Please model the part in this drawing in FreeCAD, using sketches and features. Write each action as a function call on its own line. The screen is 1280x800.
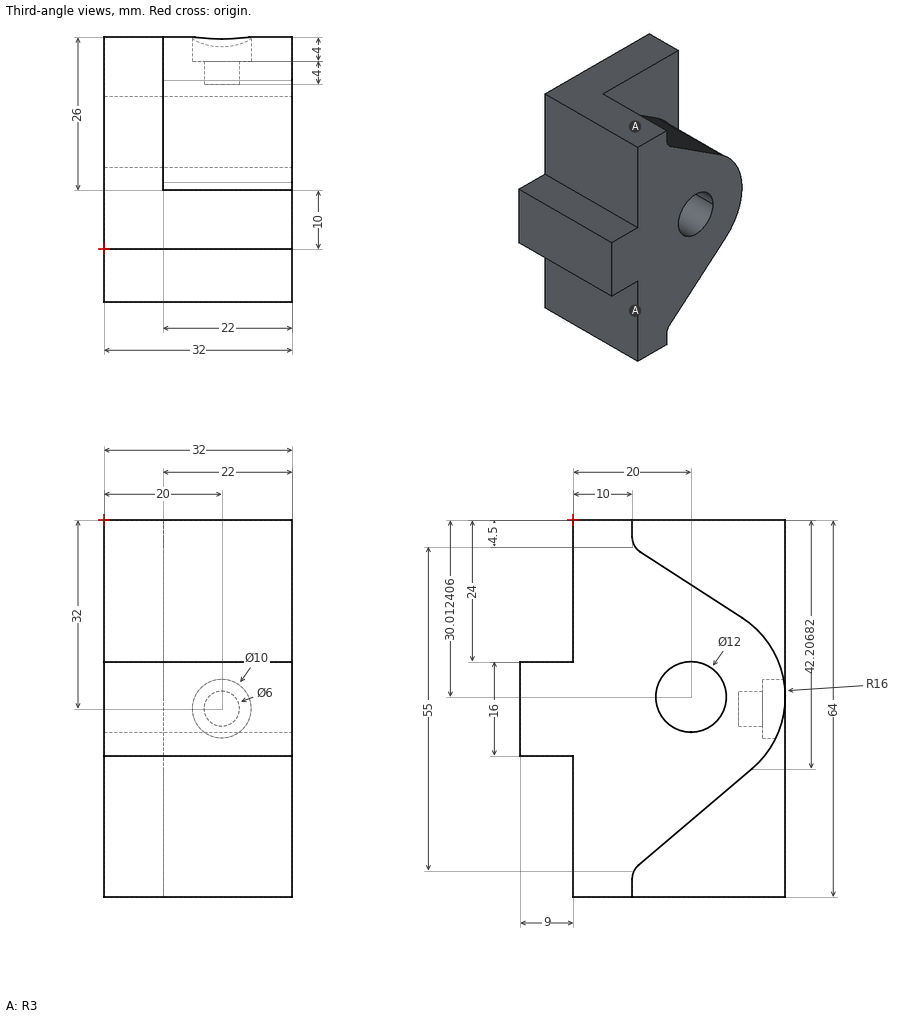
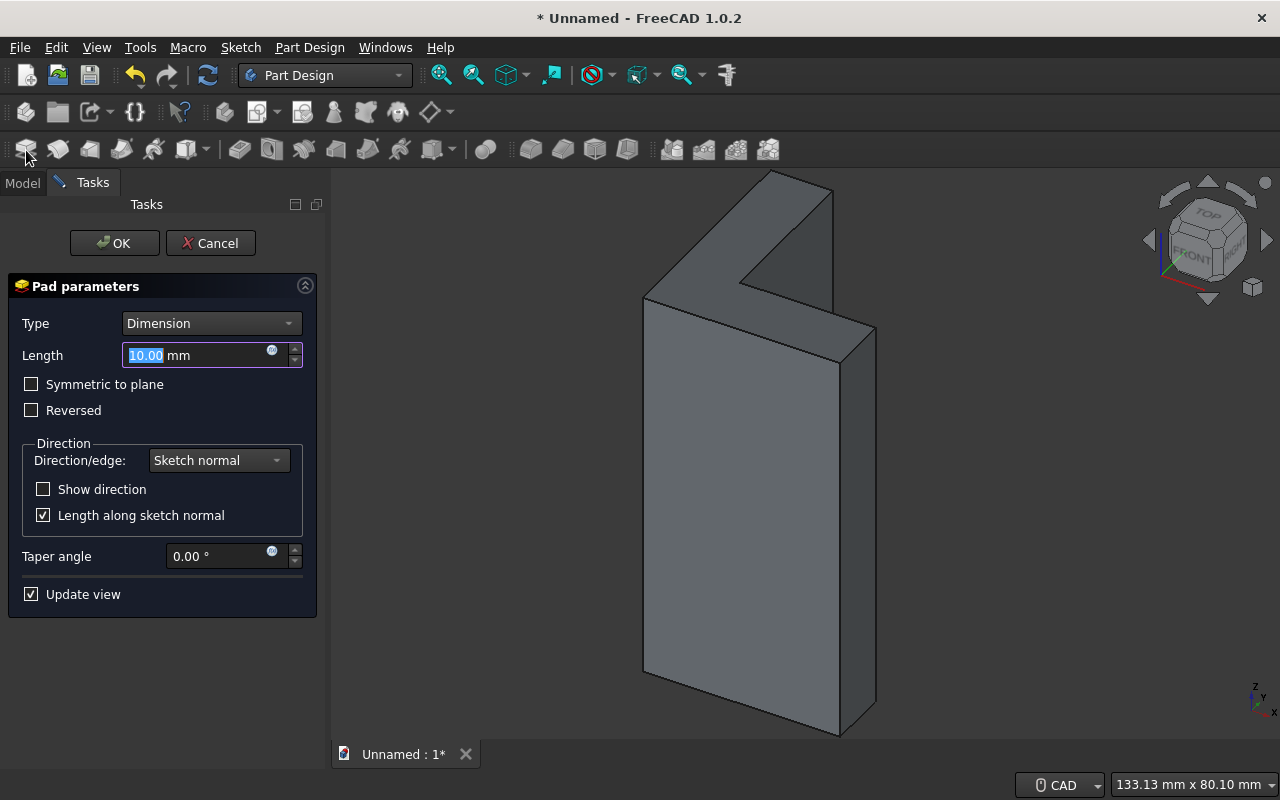
text(22)
key(Tab)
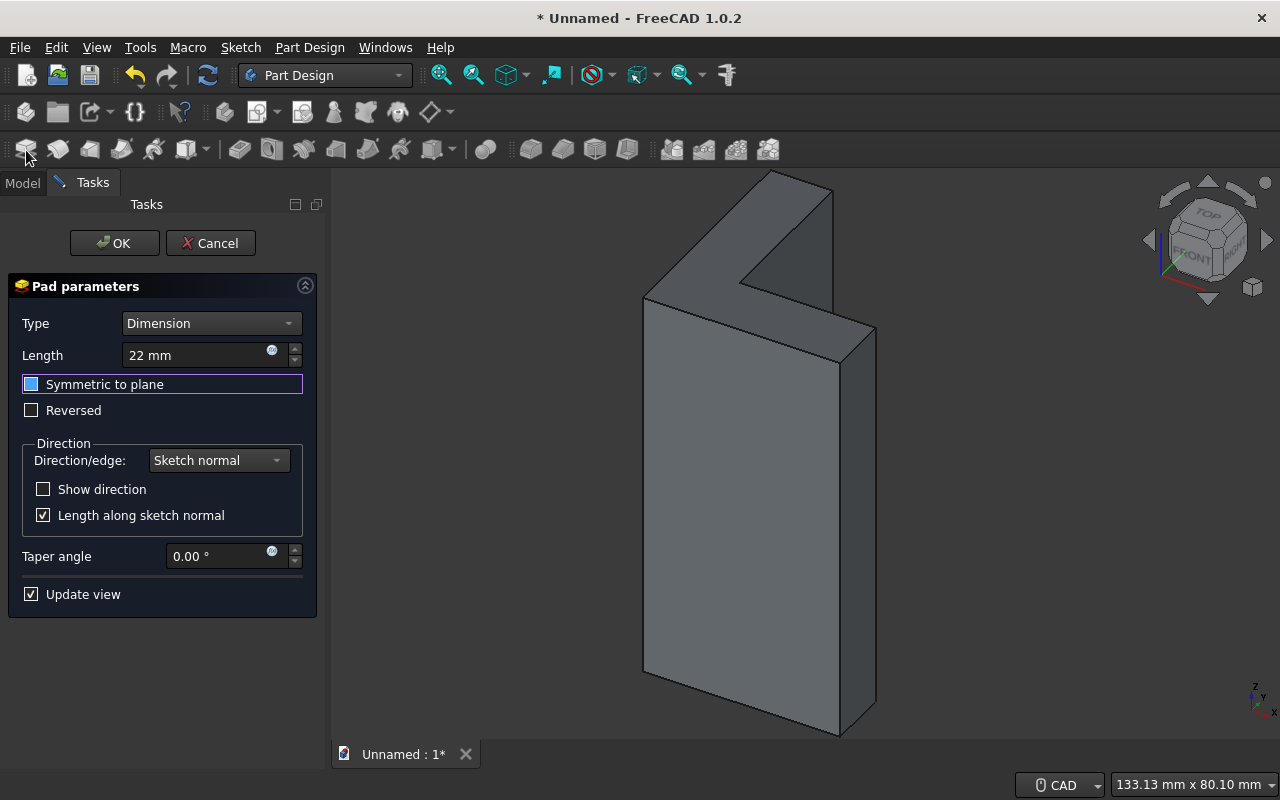
click(30, 410)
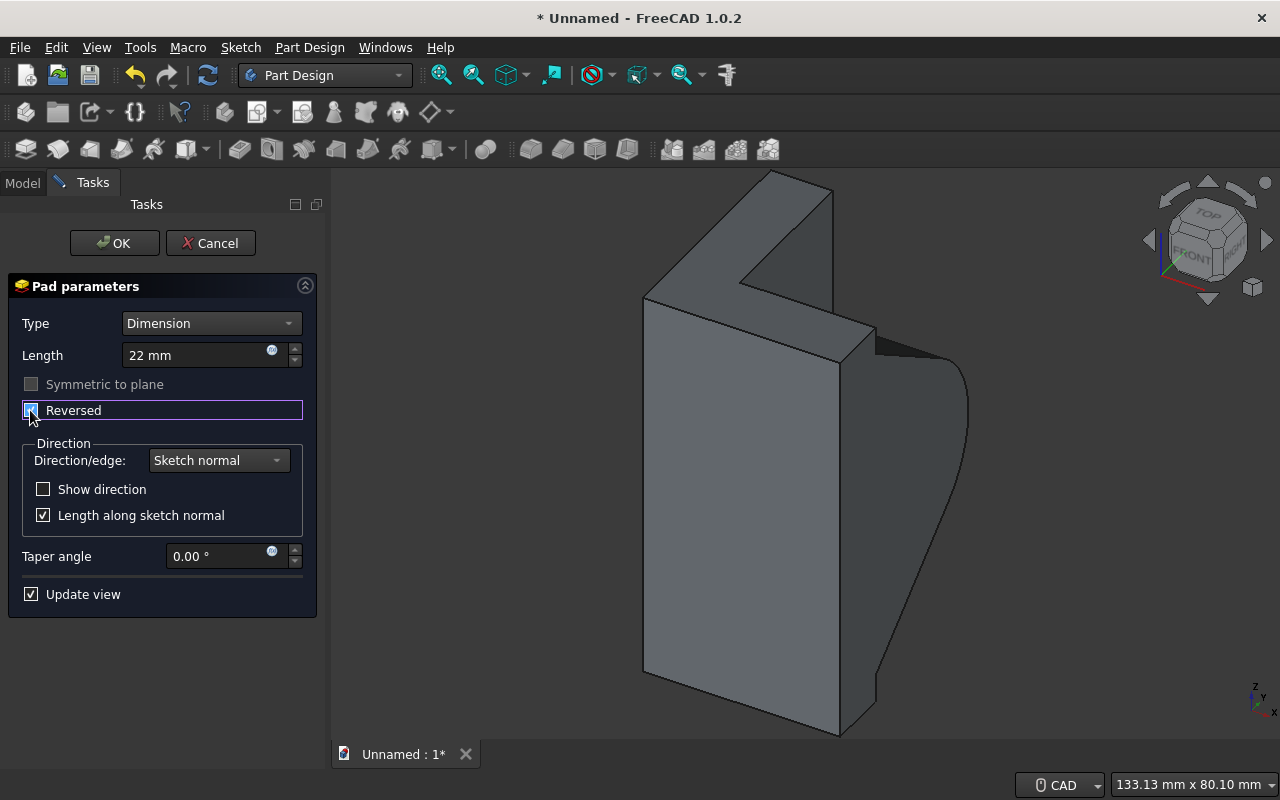
click(115, 243)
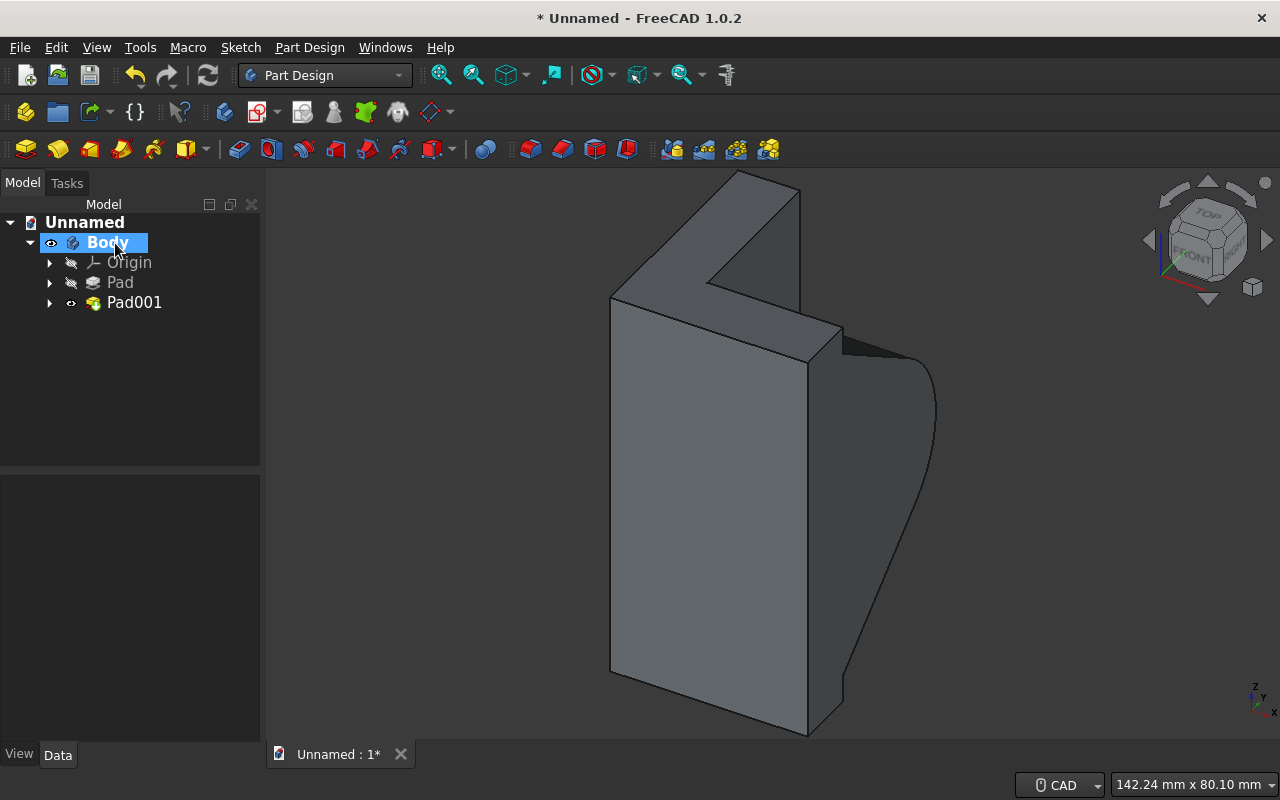
click(872, 485)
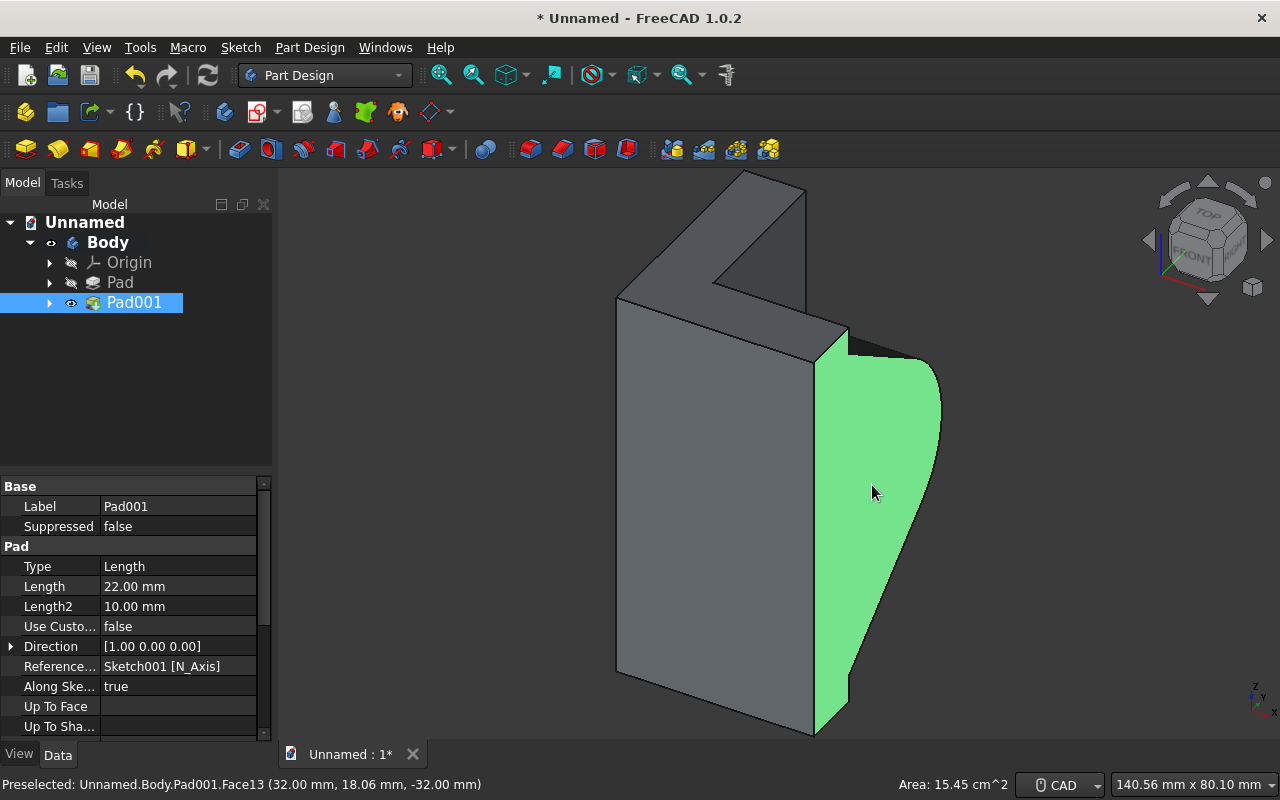
click(258, 112)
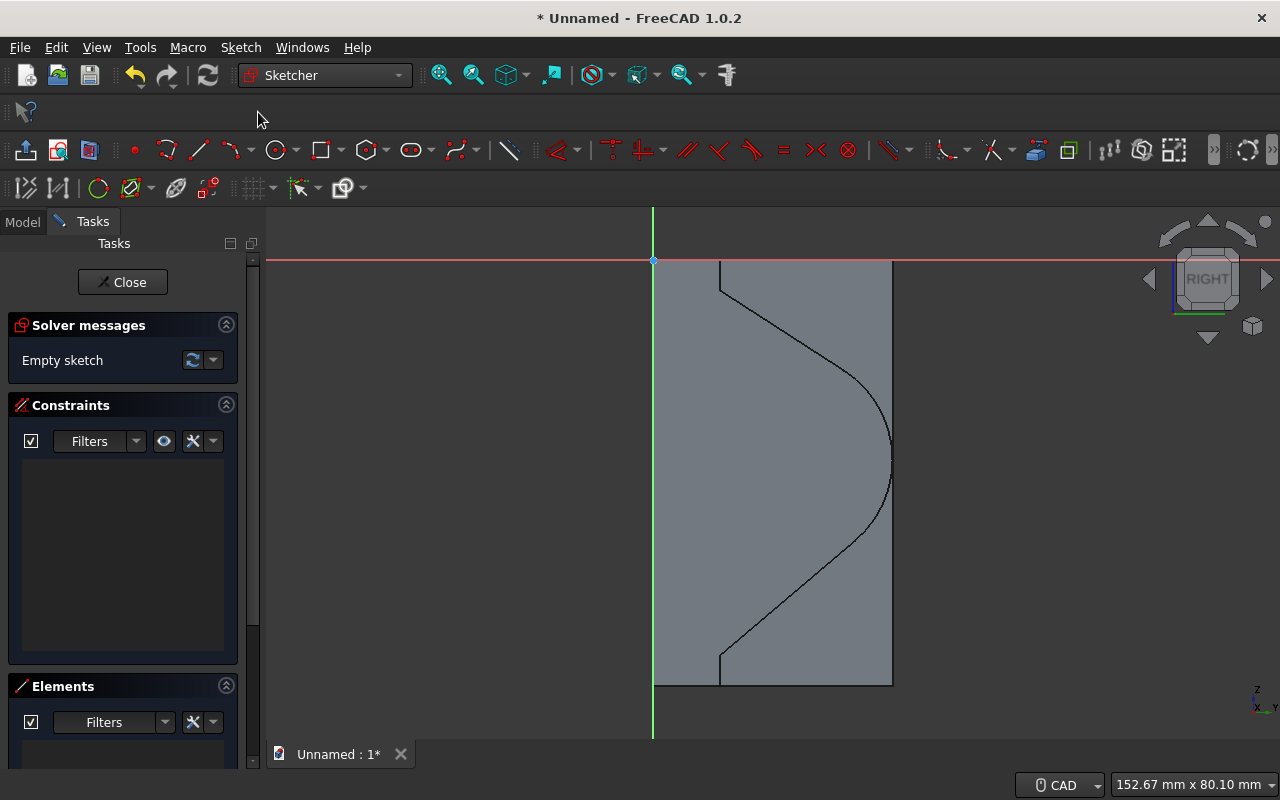
scroll(813, 455, up, 7)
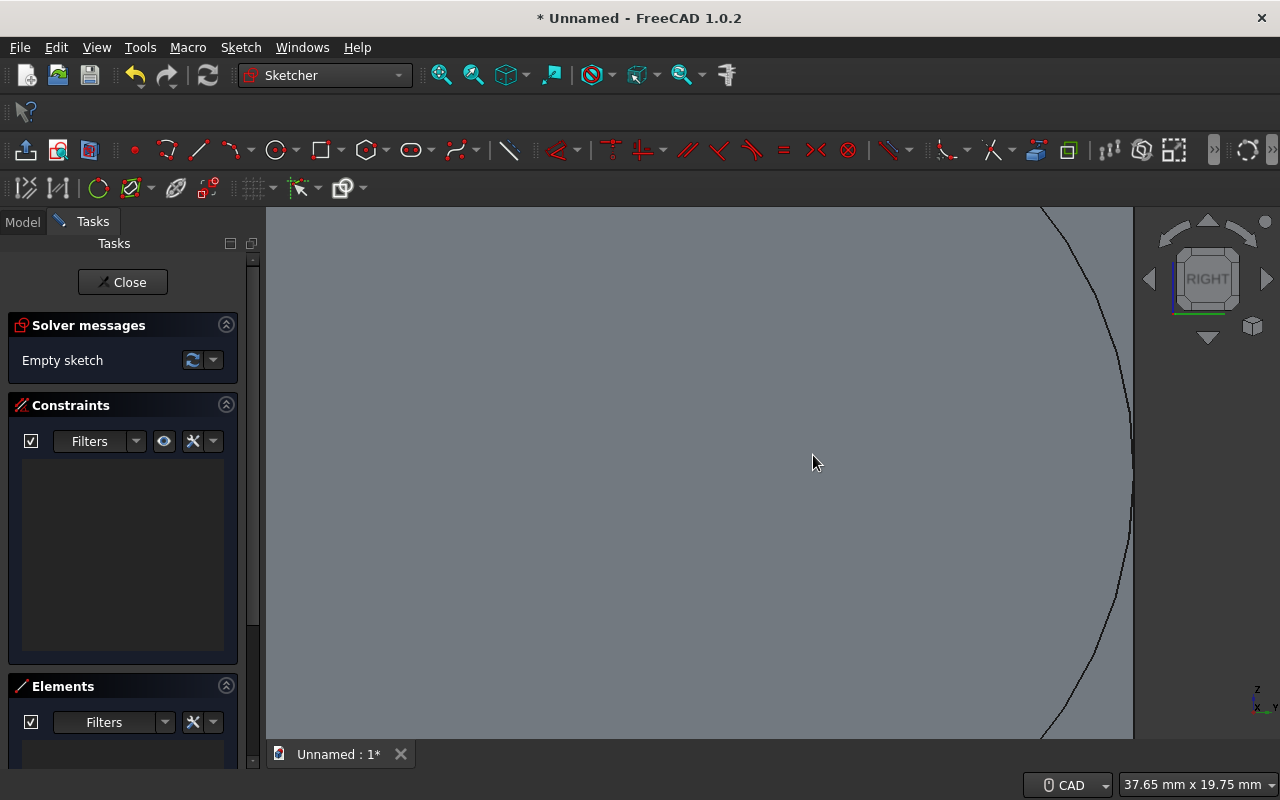
key(g)
key(c)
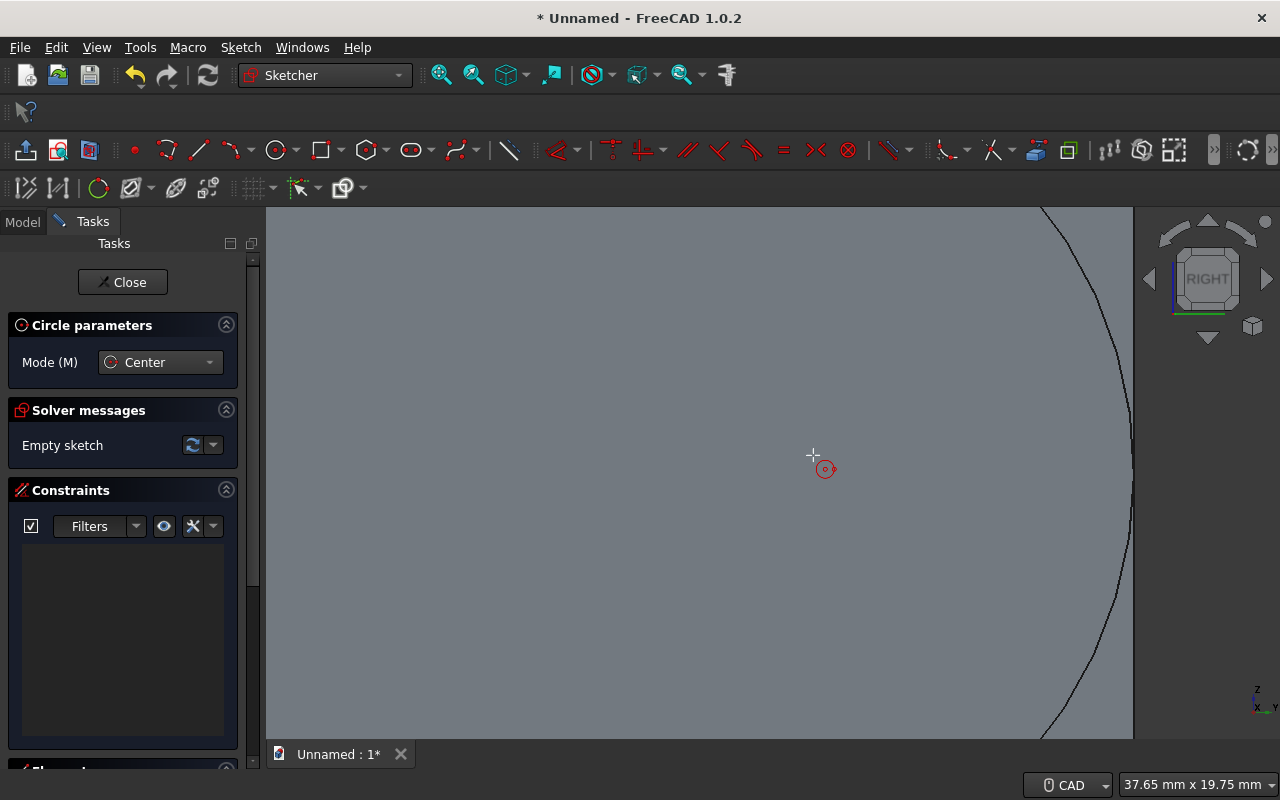
click(703, 473)
move(817, 359)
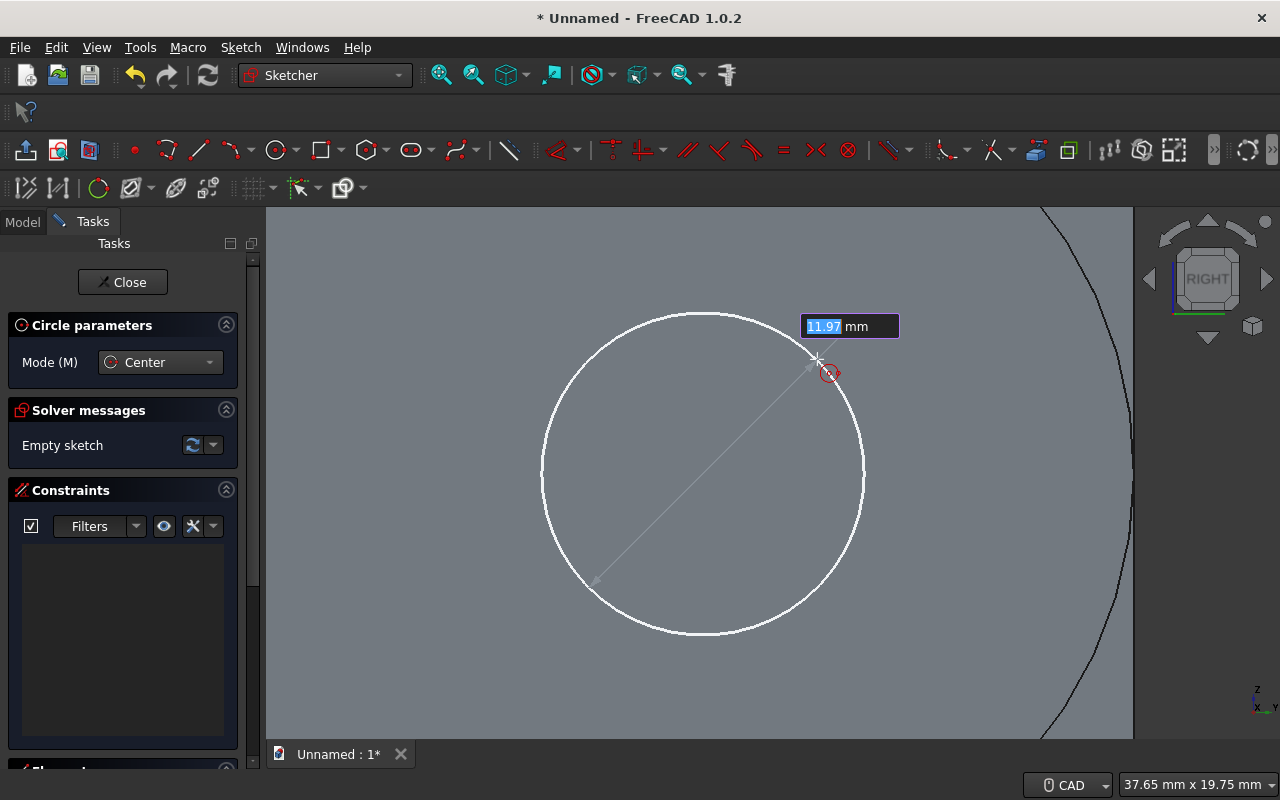
text(12)
key(Return)
key(Escape)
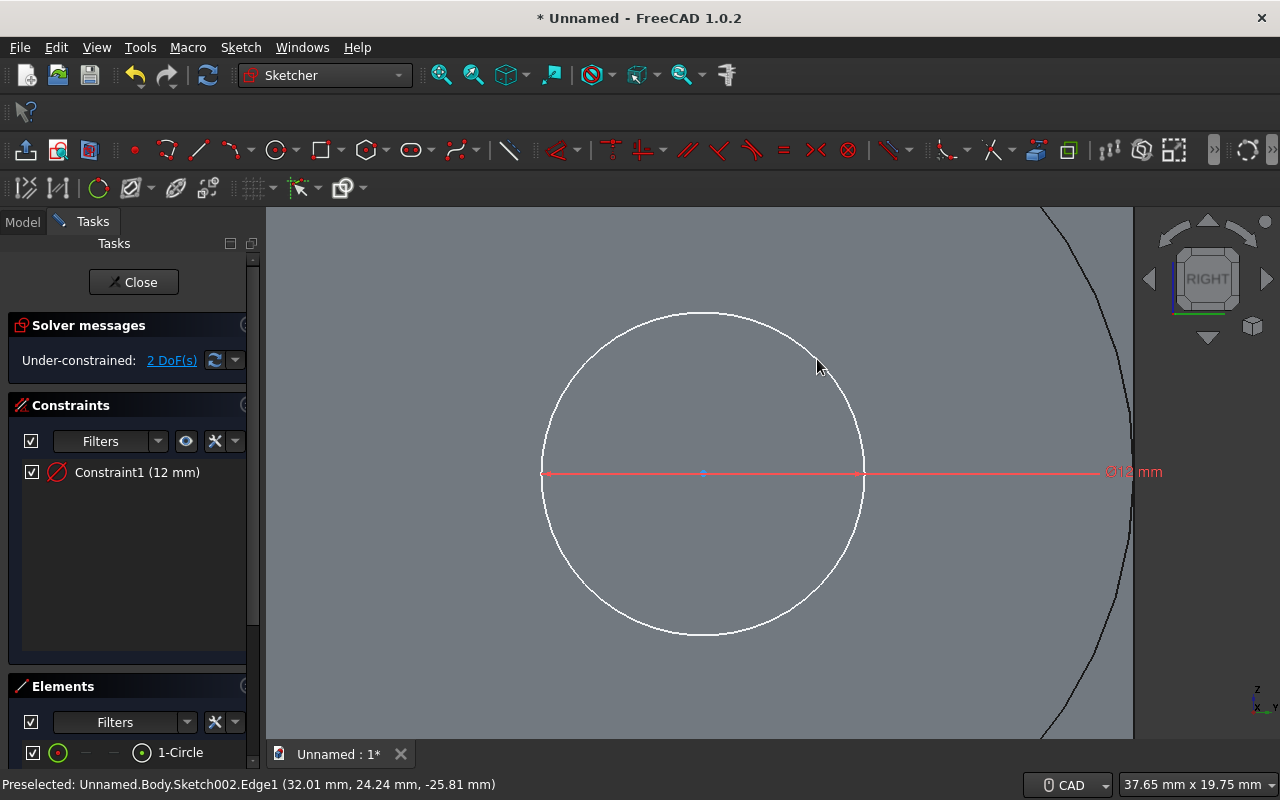
click(556, 150)